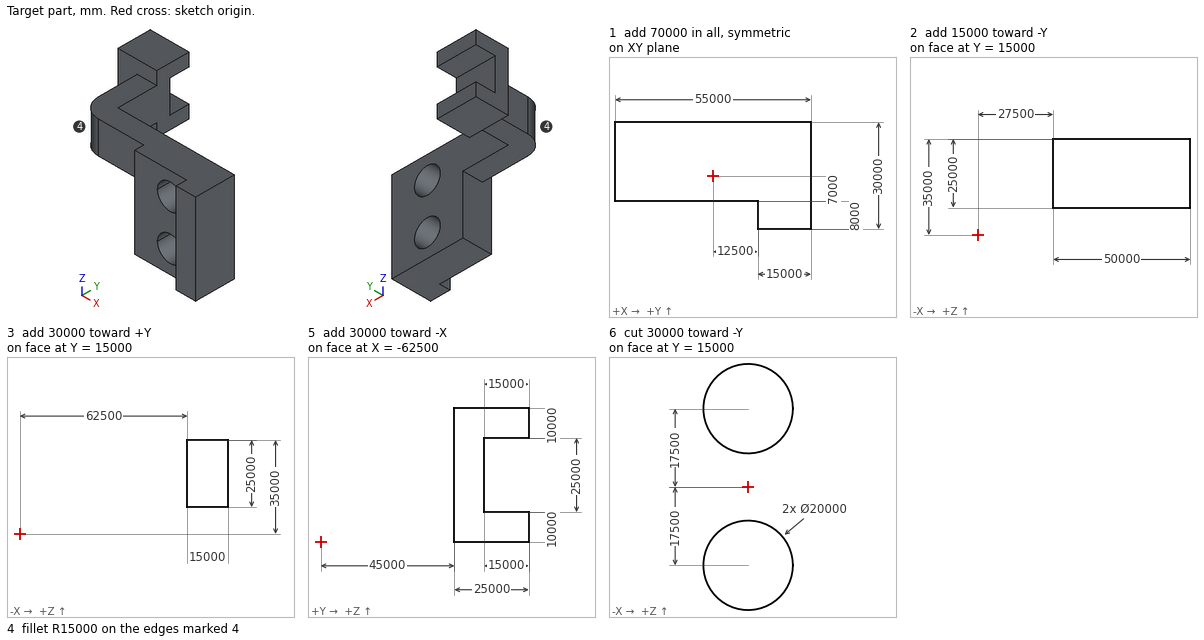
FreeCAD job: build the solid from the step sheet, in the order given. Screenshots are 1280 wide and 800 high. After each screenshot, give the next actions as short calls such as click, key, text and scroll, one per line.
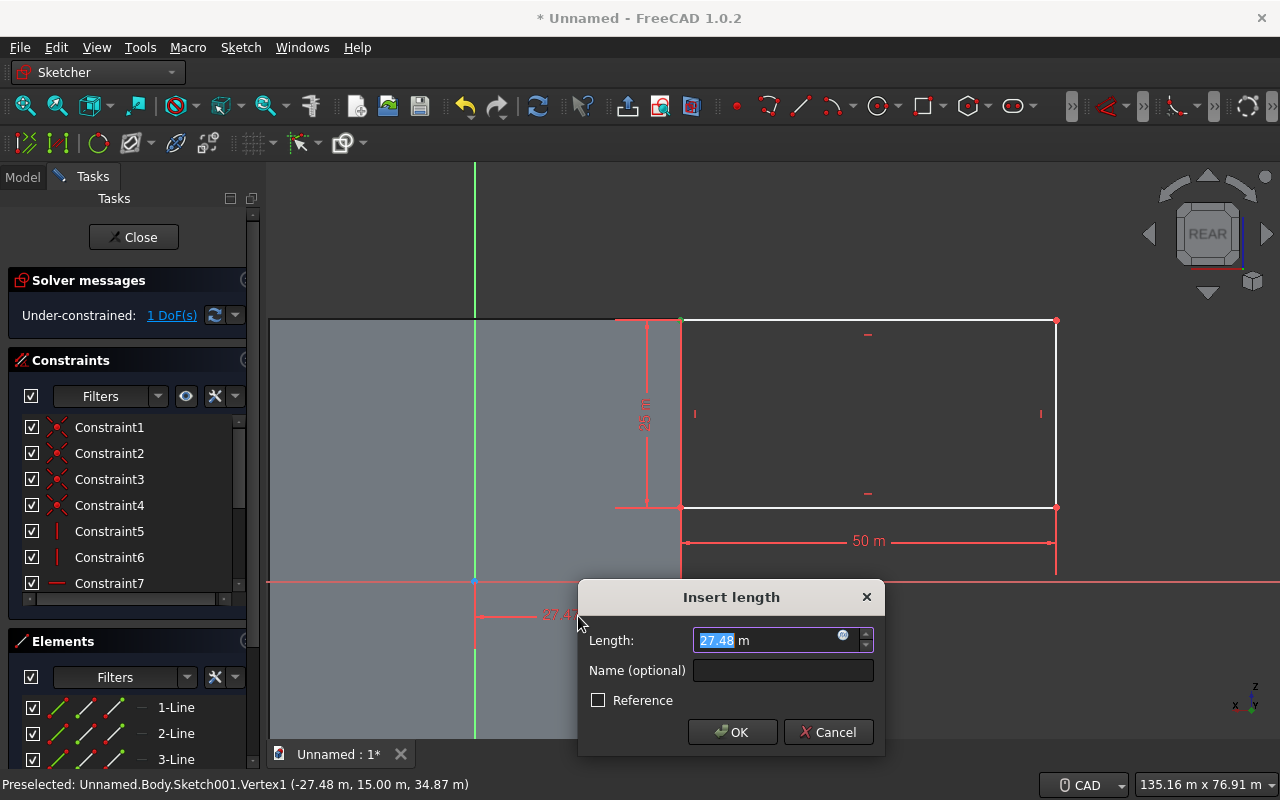
key(ctrl+a)
text(27500 mm)
key(Return)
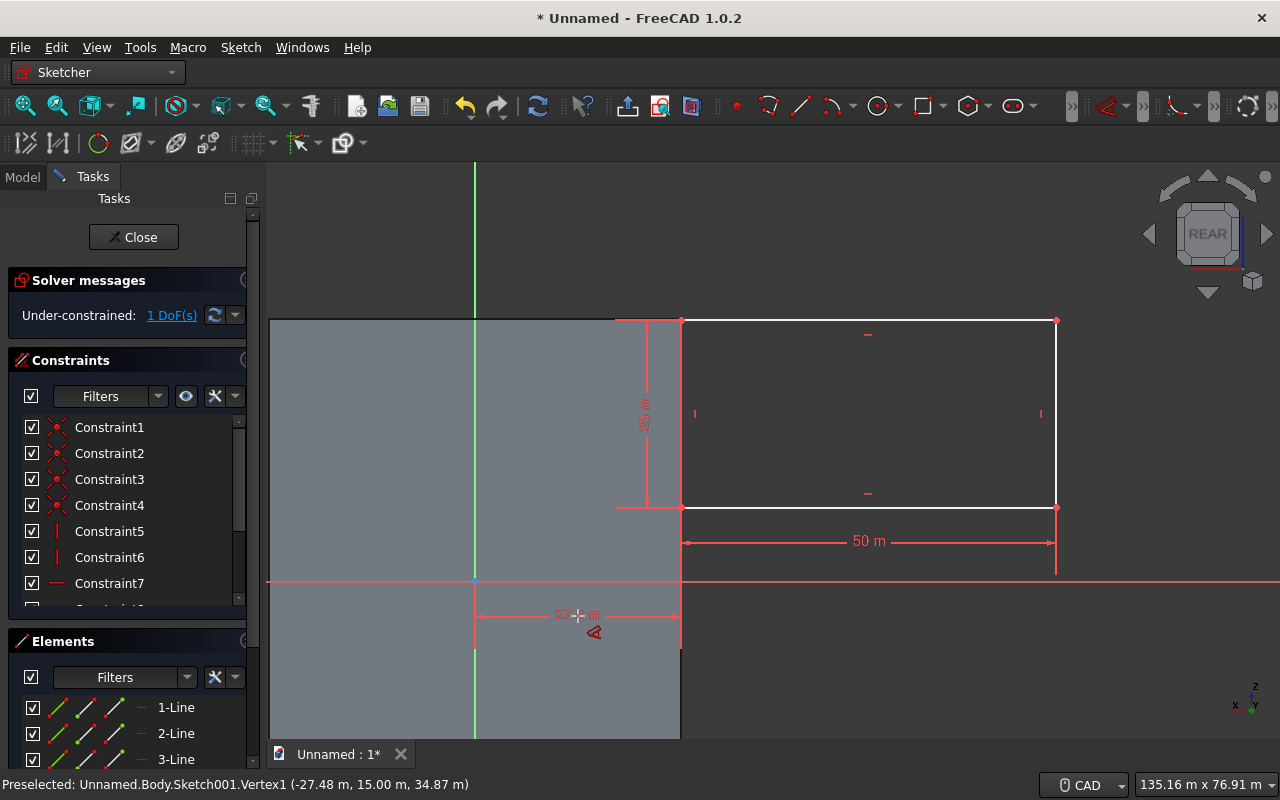
click(681, 320)
click(441, 451)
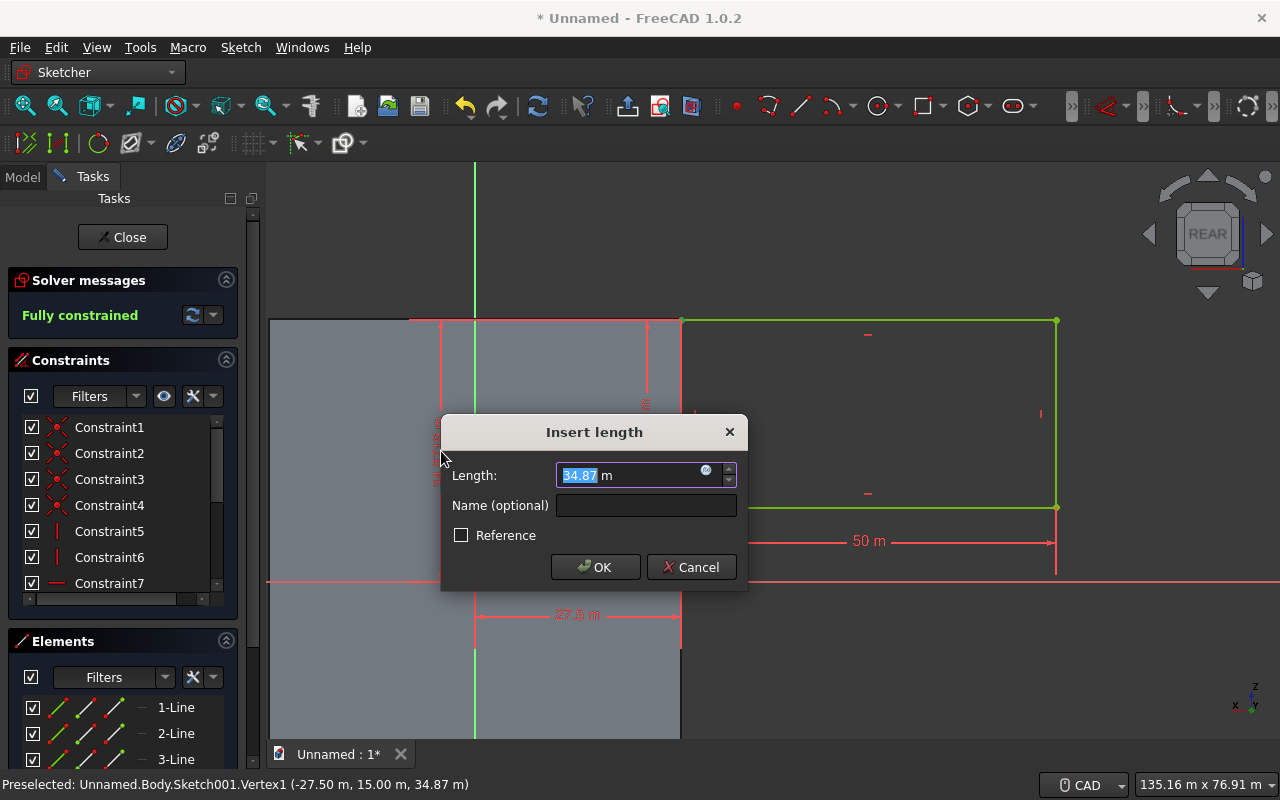
key(ctrl+a)
text(35000 mm)
key(Return)
key(Escape)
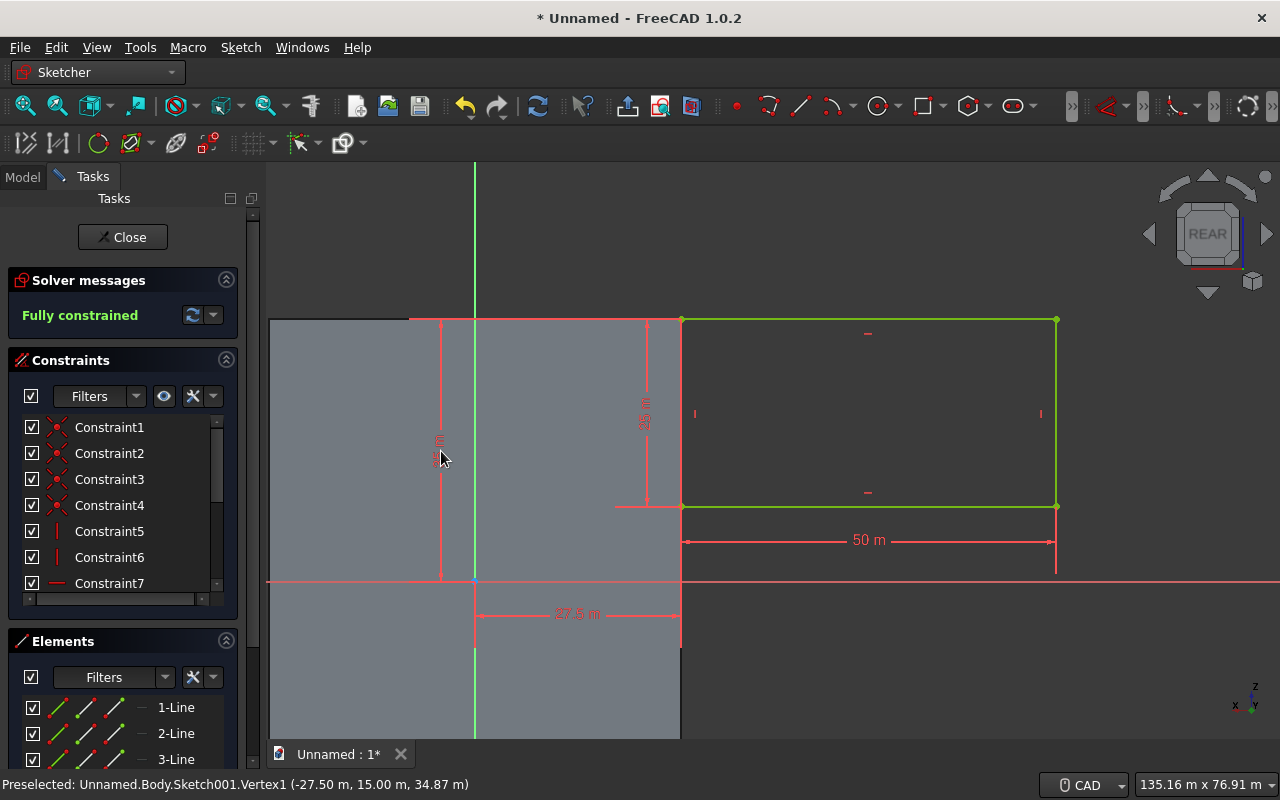
click(123, 237)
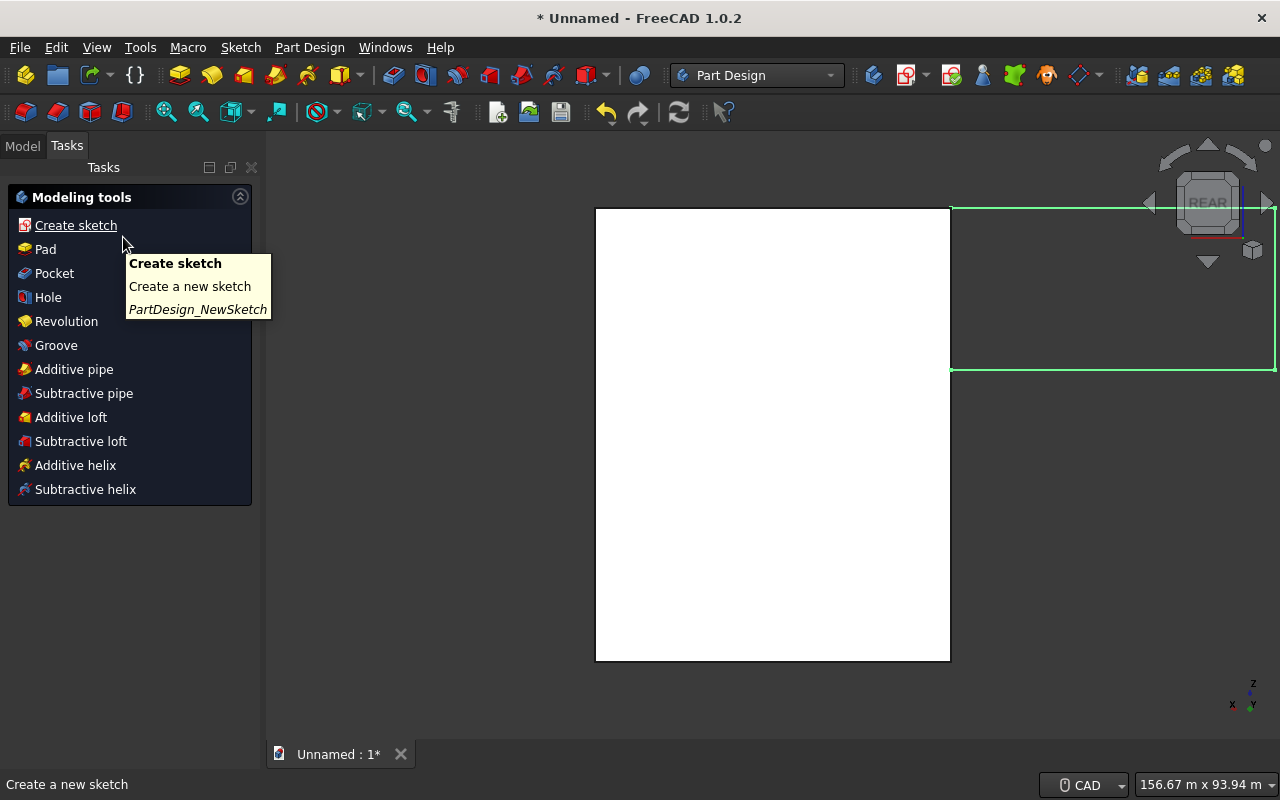
click(180, 76)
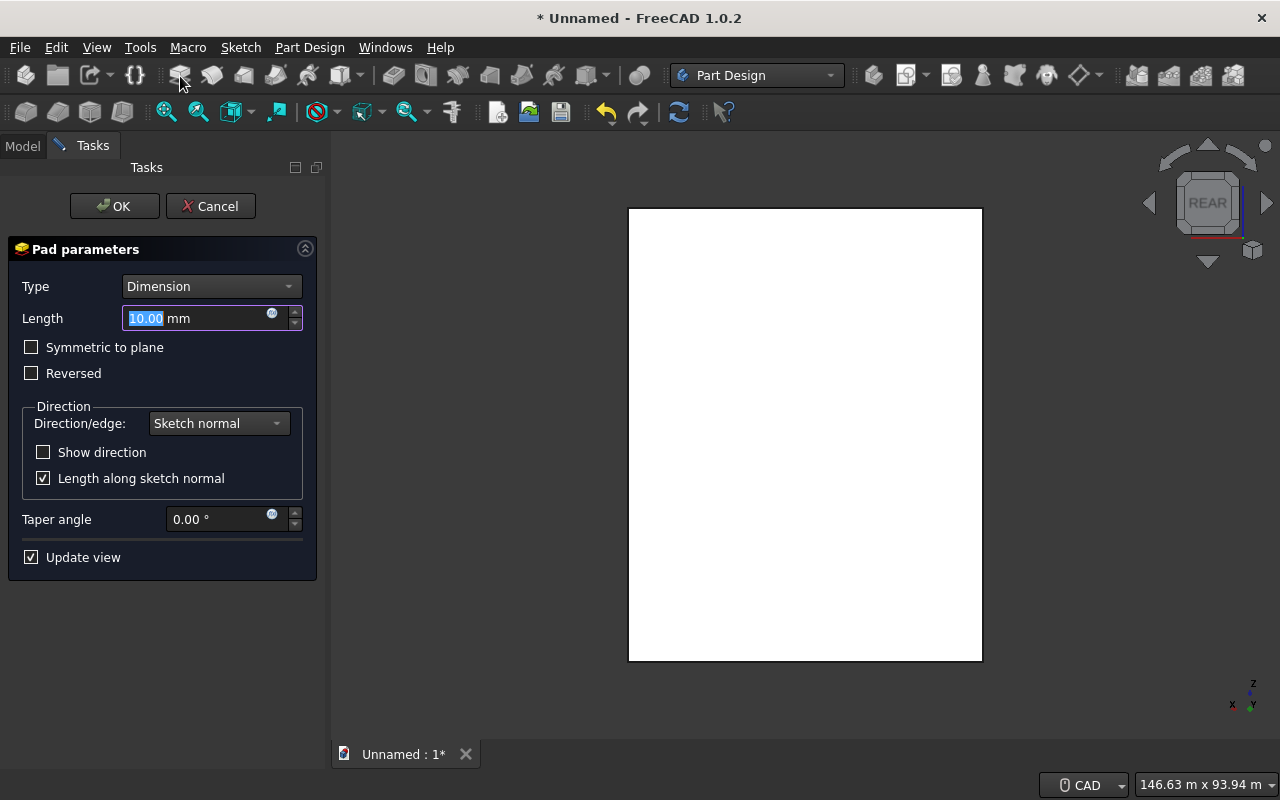
text(15000)
key(Tab)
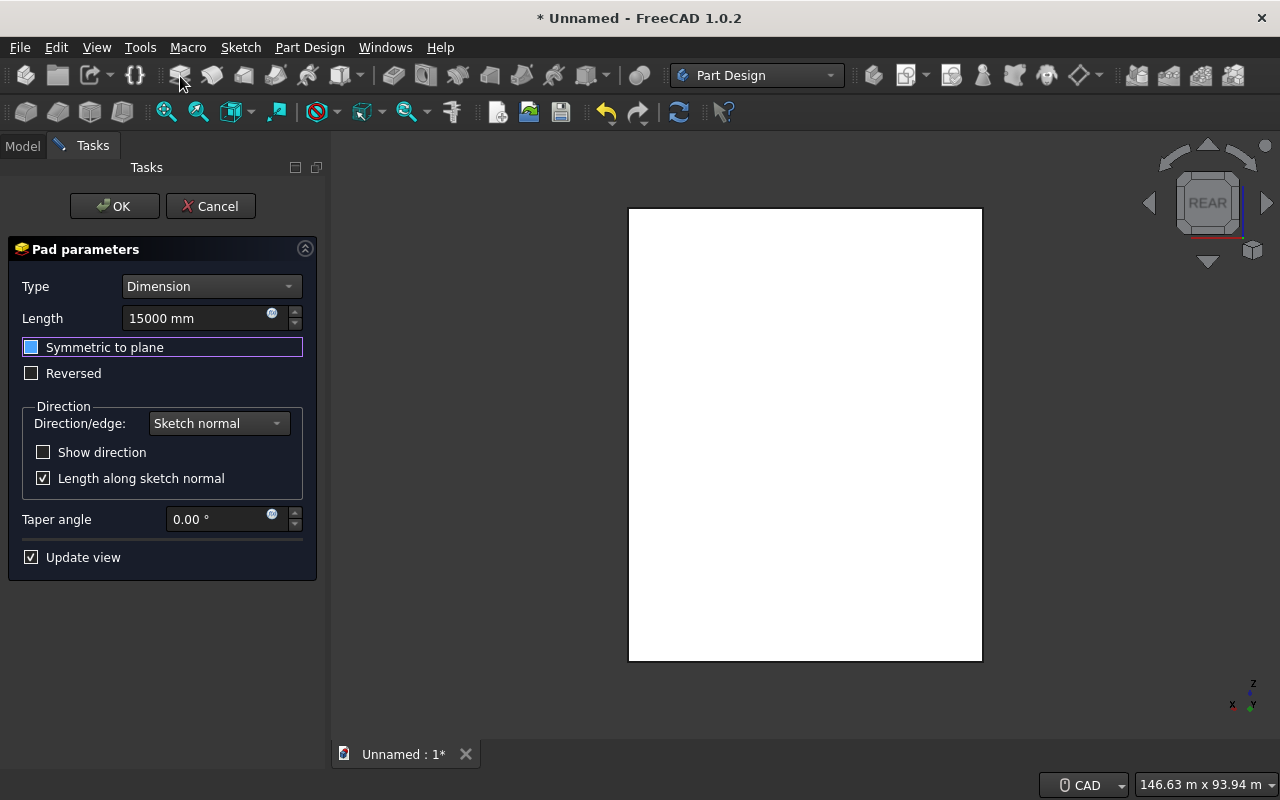
click(30, 373)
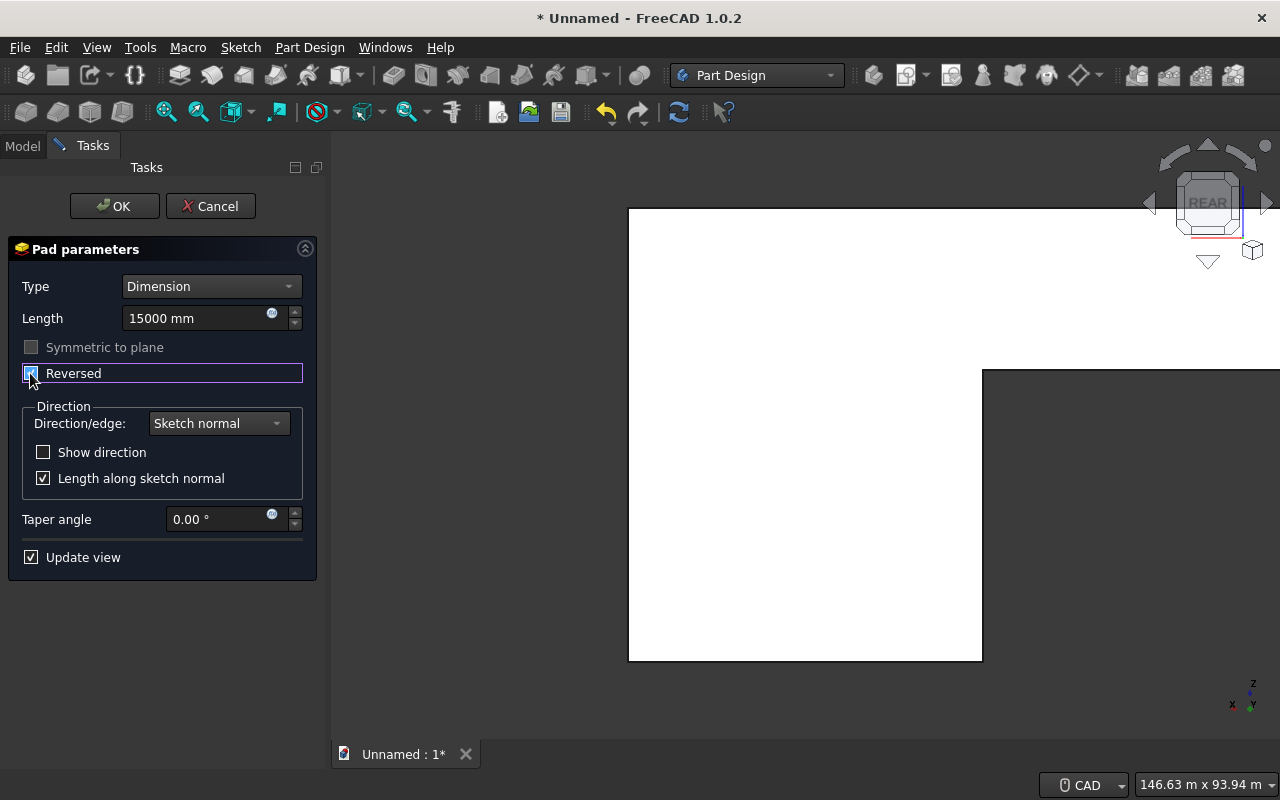
click(115, 206)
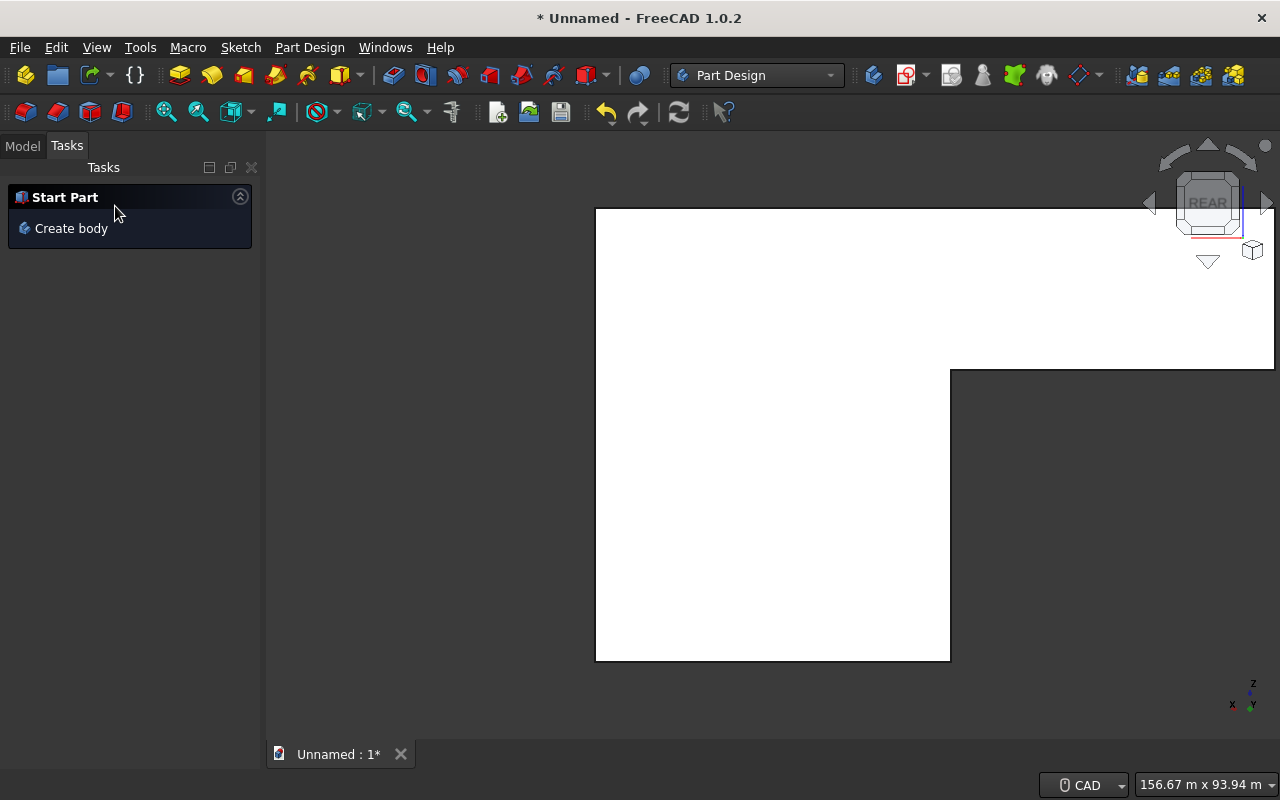
click(741, 369)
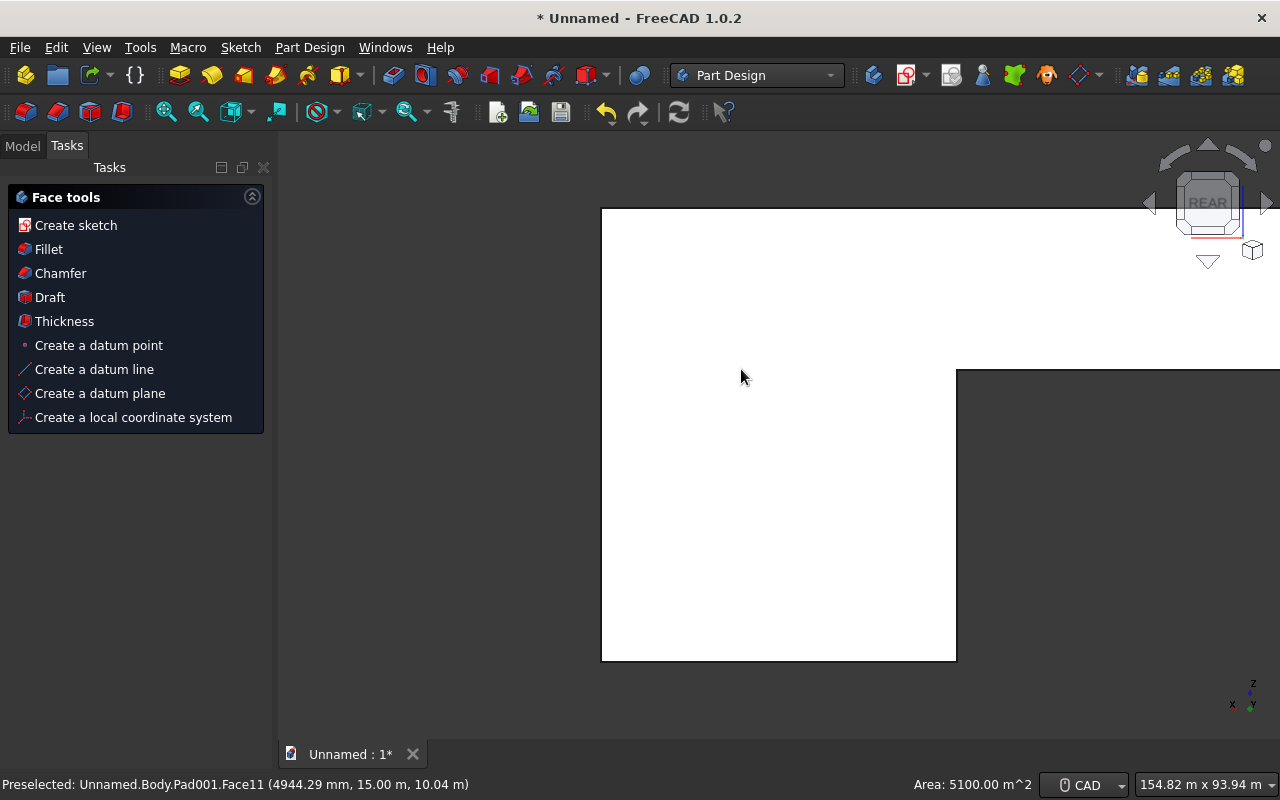
click(906, 76)